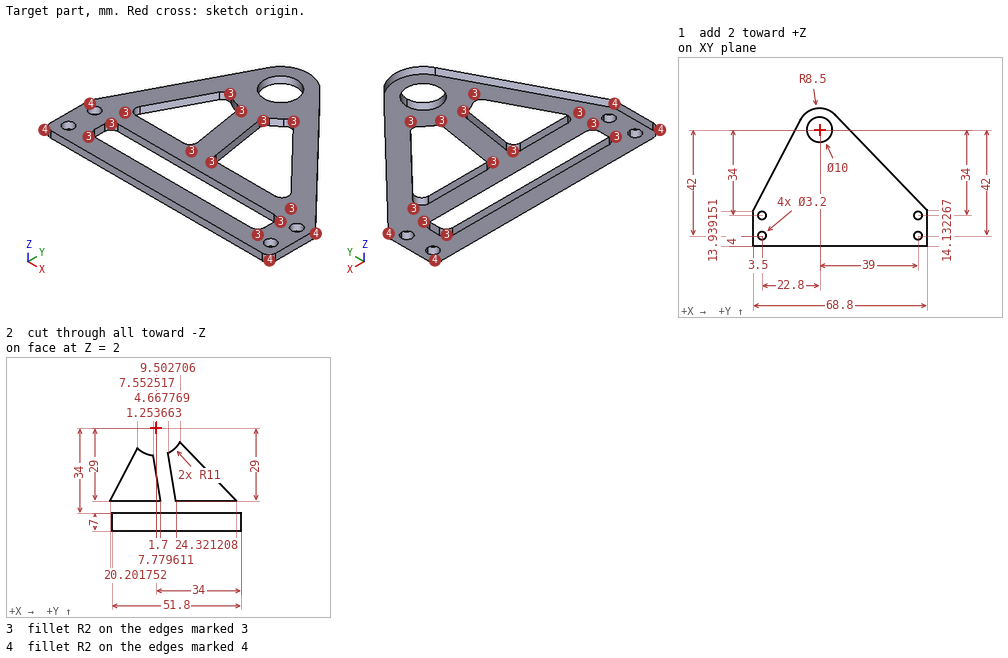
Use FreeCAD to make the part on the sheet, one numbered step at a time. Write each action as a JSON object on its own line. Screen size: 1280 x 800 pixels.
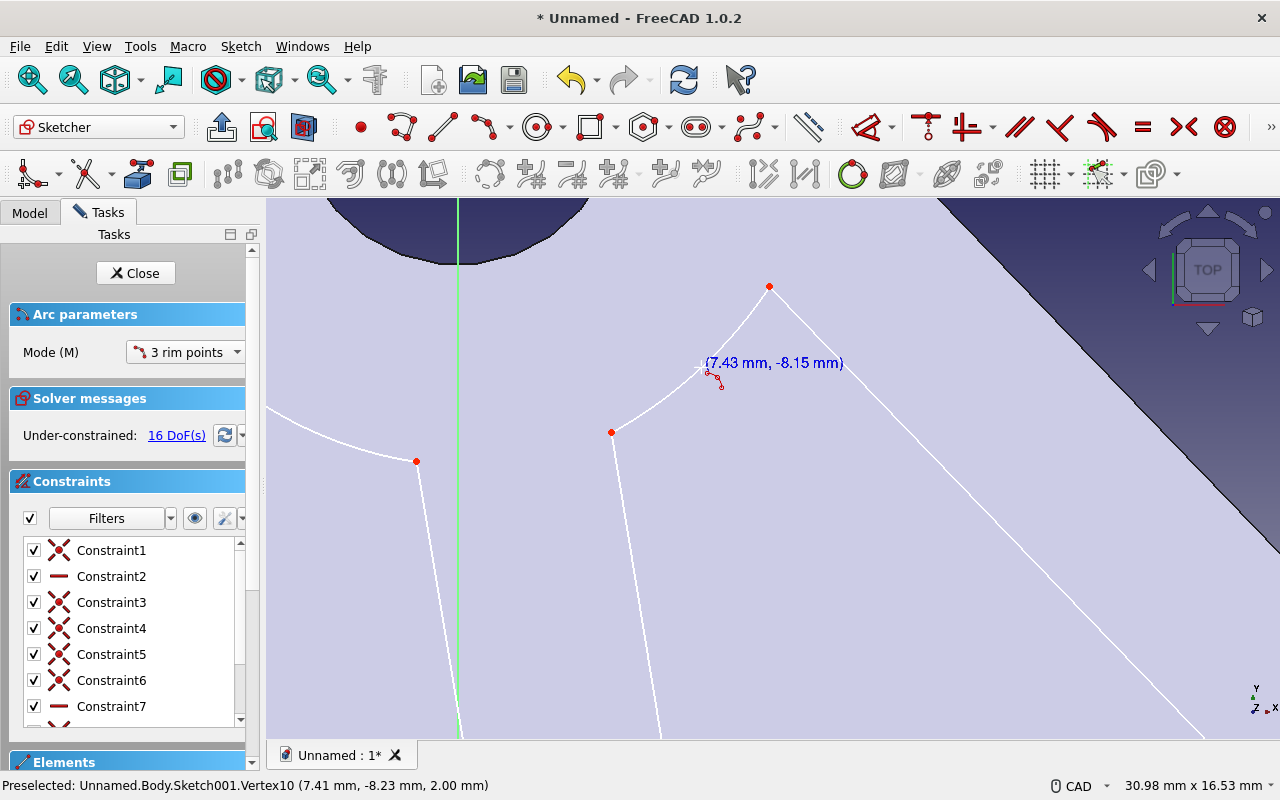
{"action": "left_click", "coordinate": [590, 128]}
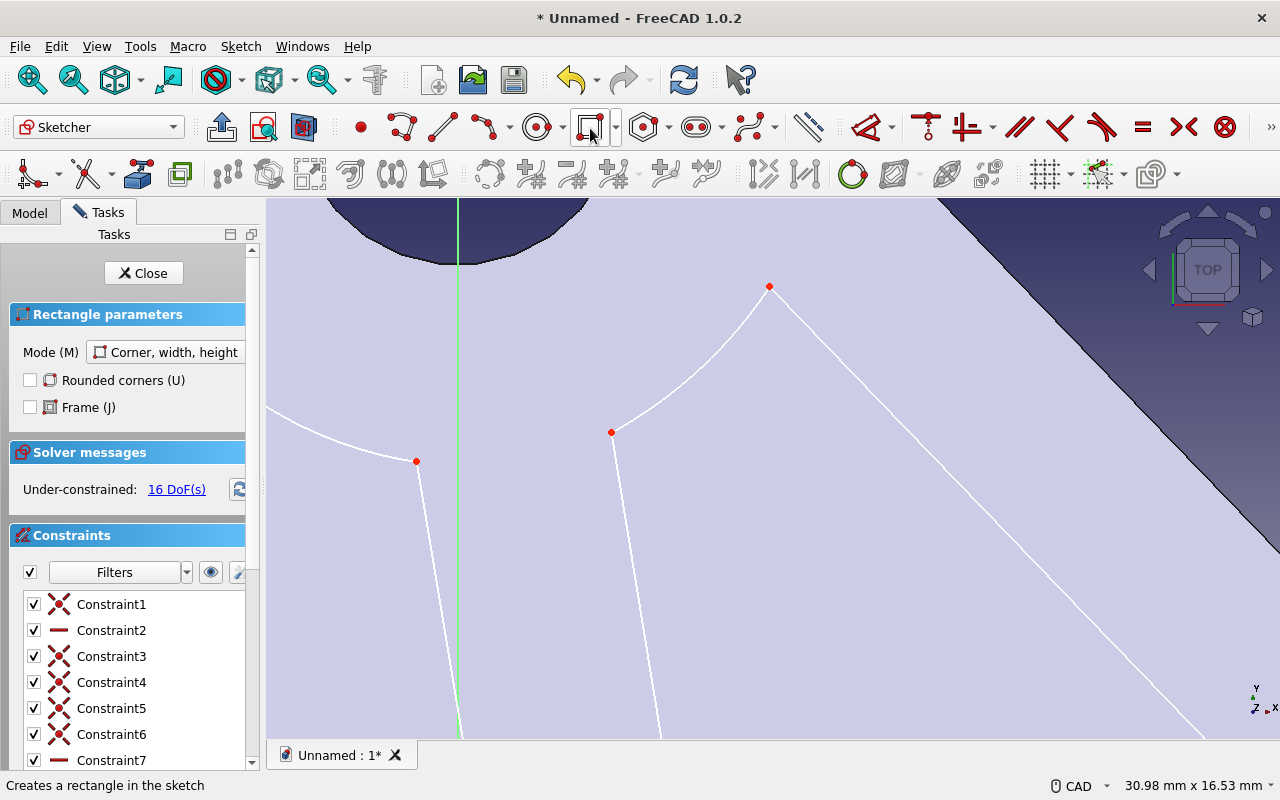
{"action": "scroll", "coordinate": [702, 369], "scroll_direction": "down", "scroll_amount": 7}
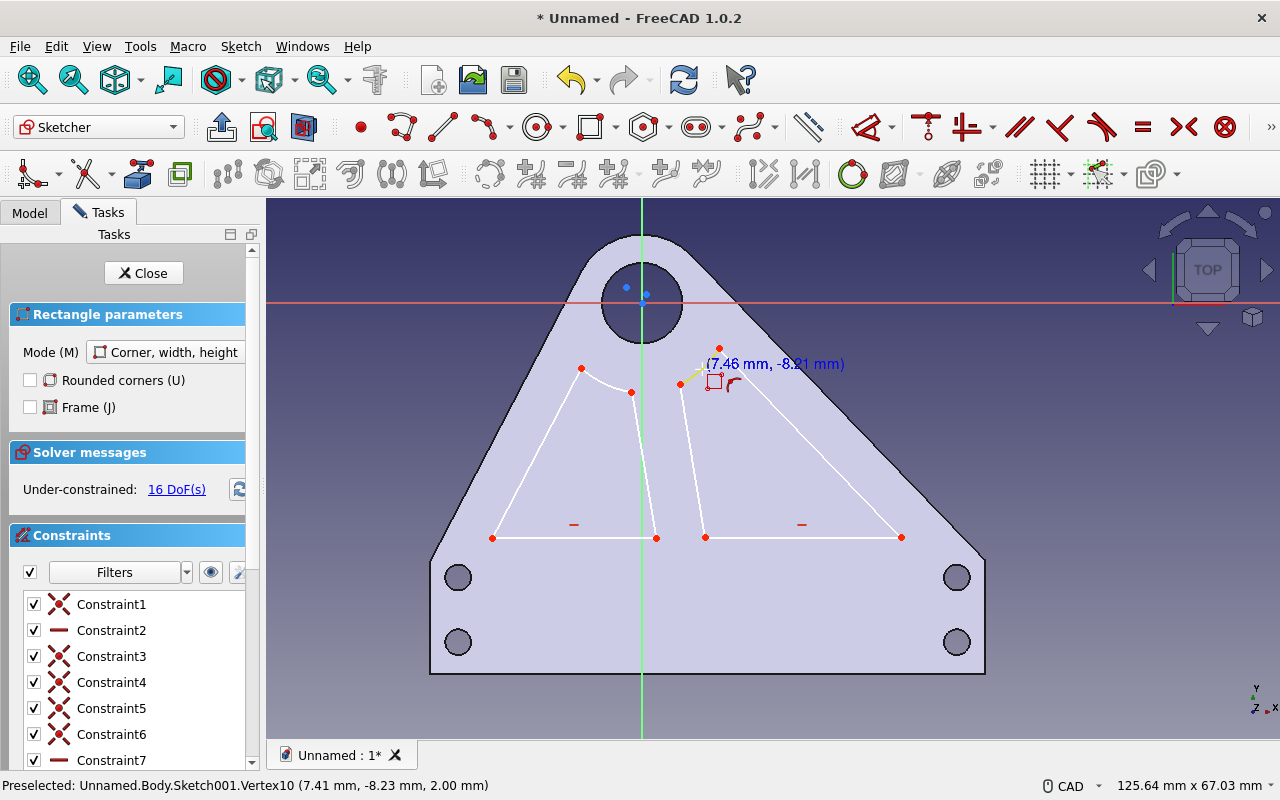
{"action": "left_click", "coordinate": [498, 578]}
{"action": "left_click", "coordinate": [917, 634]}
{"action": "key", "text": "Escape"}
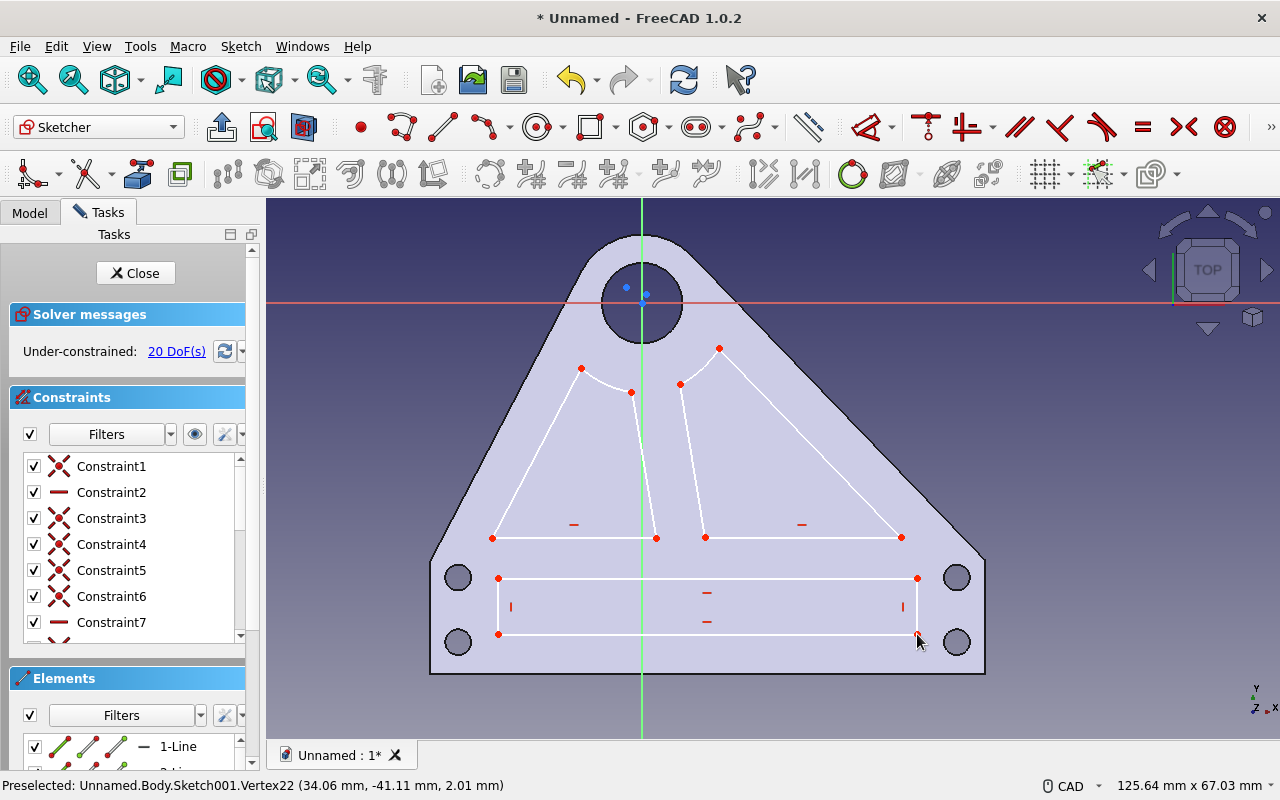
{"action": "left_click", "coordinate": [595, 379]}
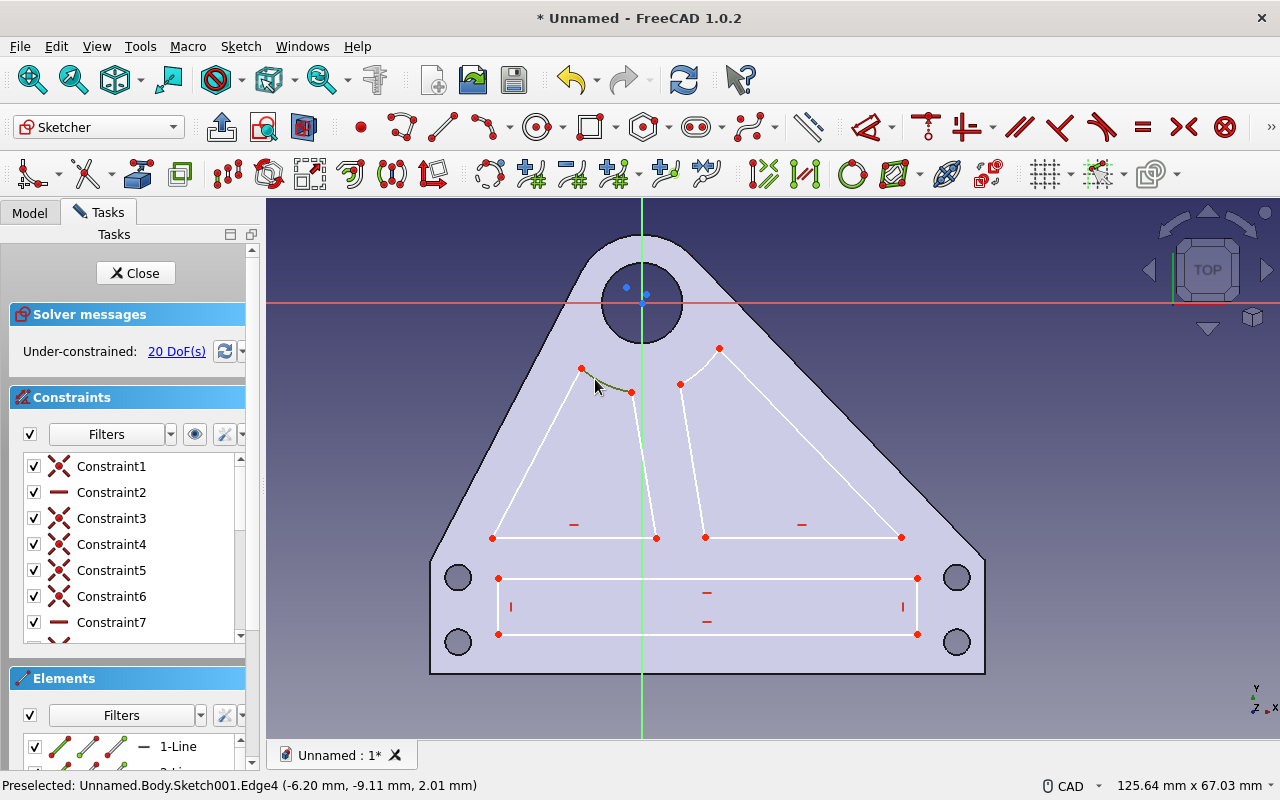
{"action": "left_click", "coordinate": [693, 376]}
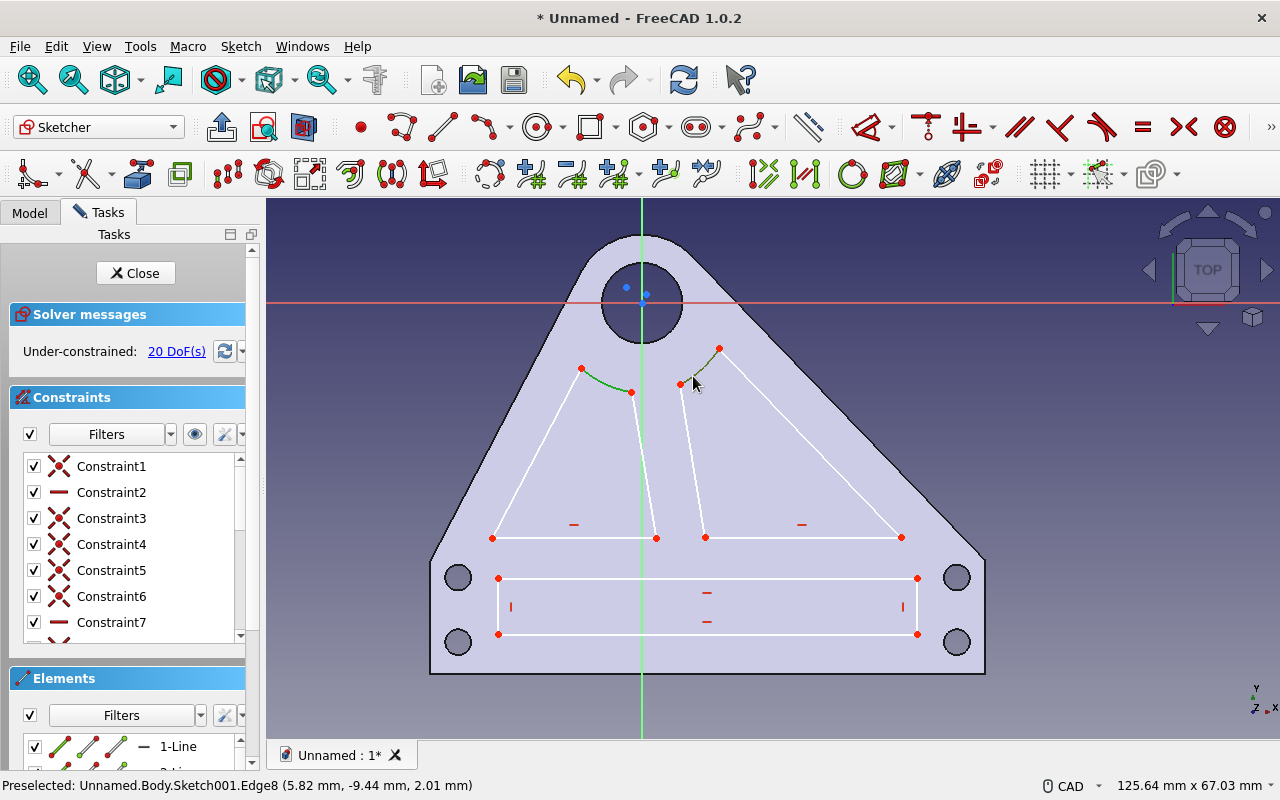
{"action": "key", "text": "c"}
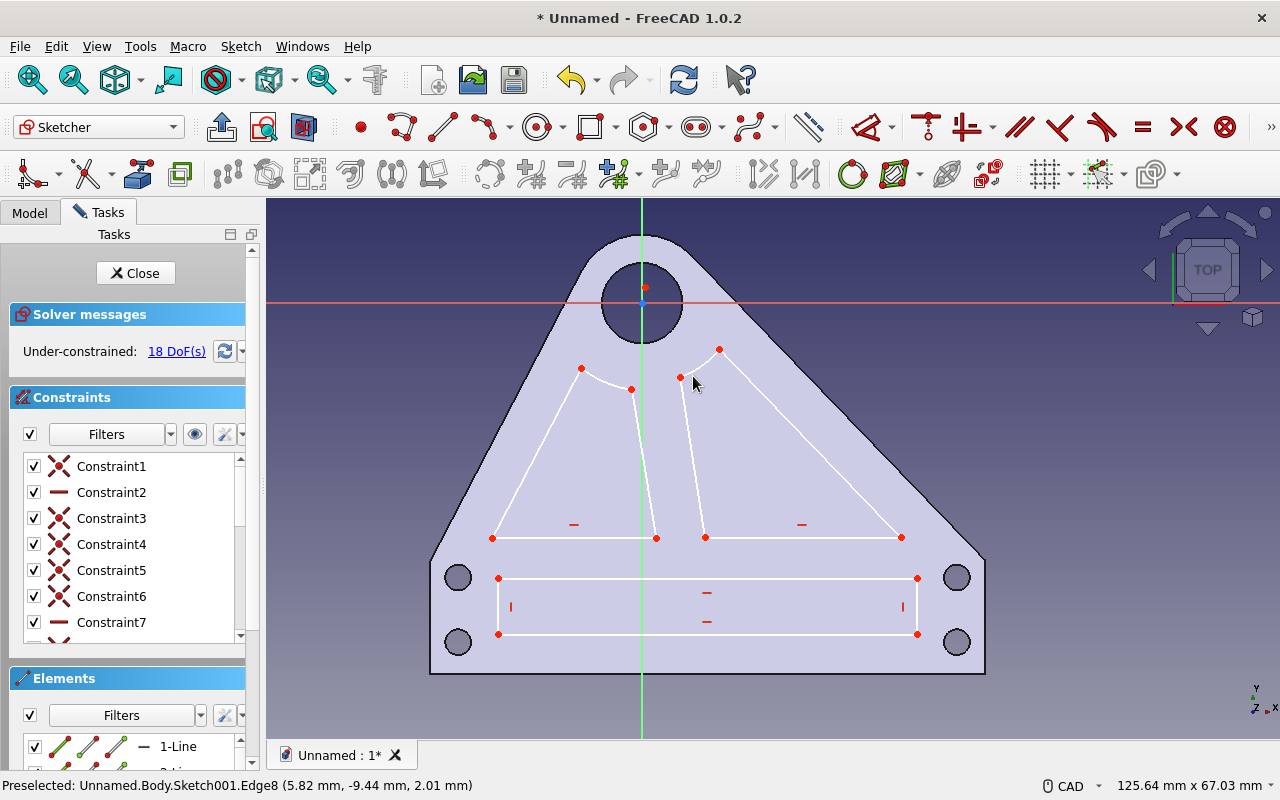
{"action": "left_click_drag", "start_coordinate": [632, 277], "coordinate": [656, 313]}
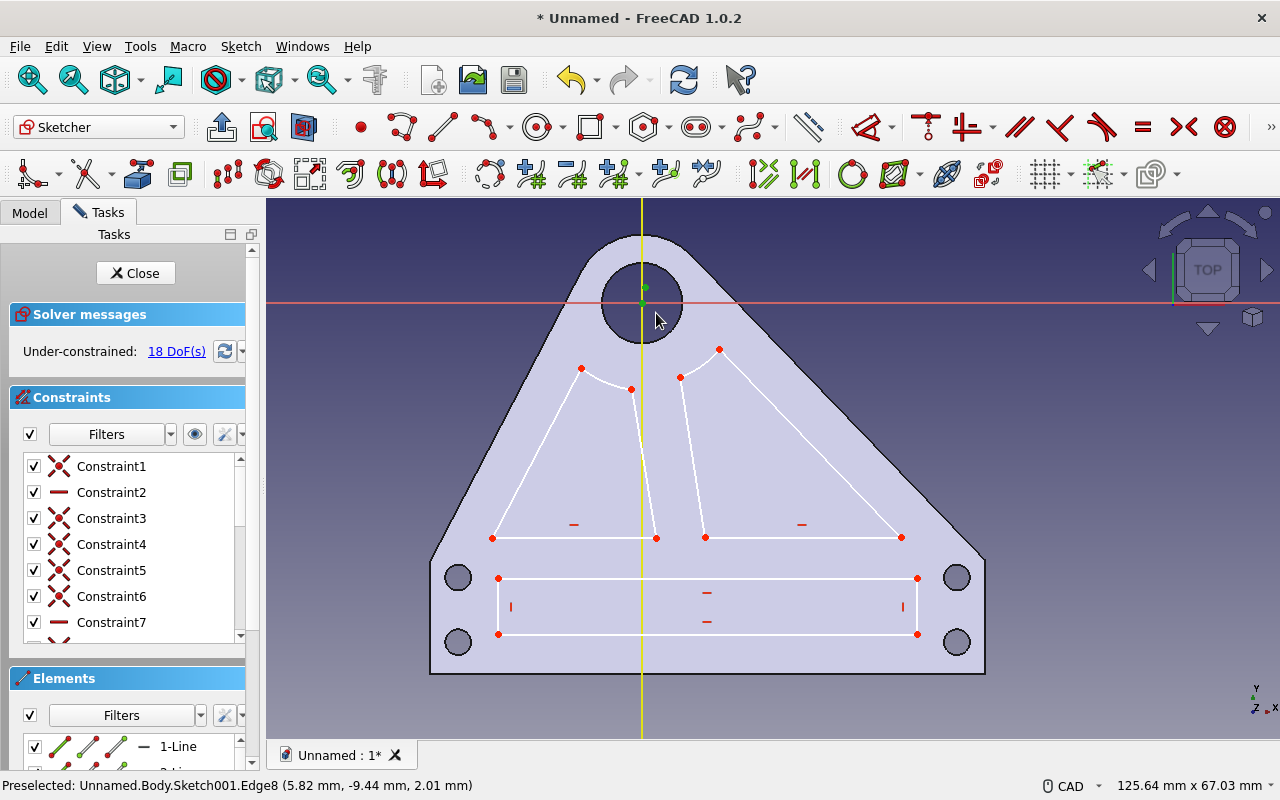
{"action": "left_click", "coordinate": [926, 128]}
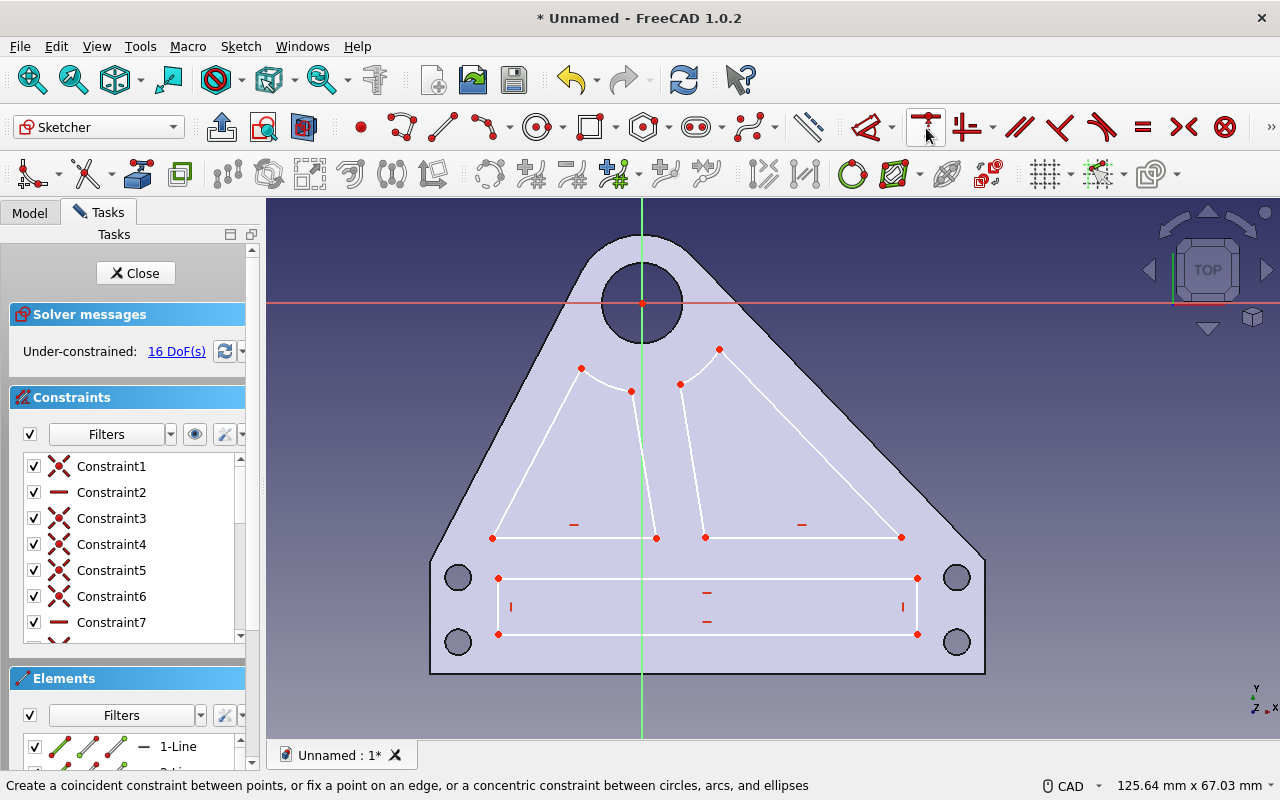
{"action": "left_click", "coordinate": [595, 379]}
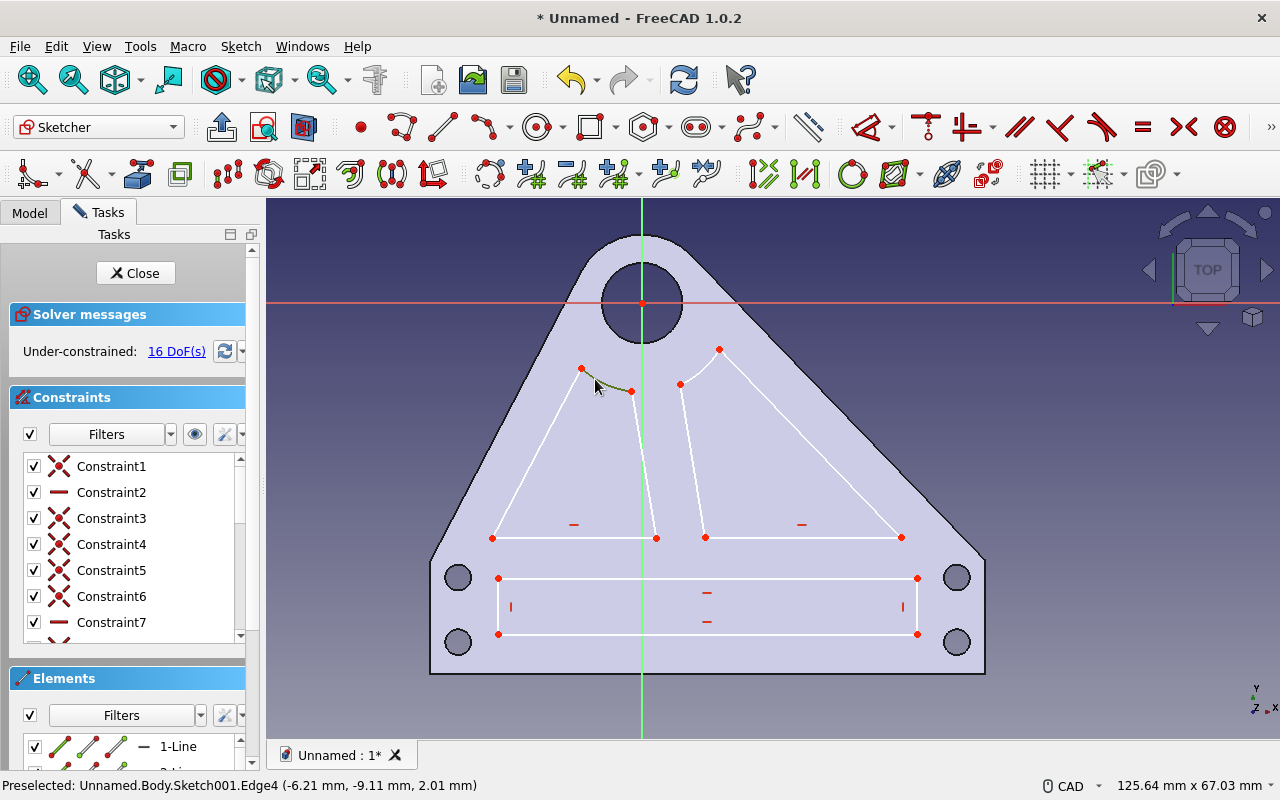
{"action": "left_click", "coordinate": [694, 377]}